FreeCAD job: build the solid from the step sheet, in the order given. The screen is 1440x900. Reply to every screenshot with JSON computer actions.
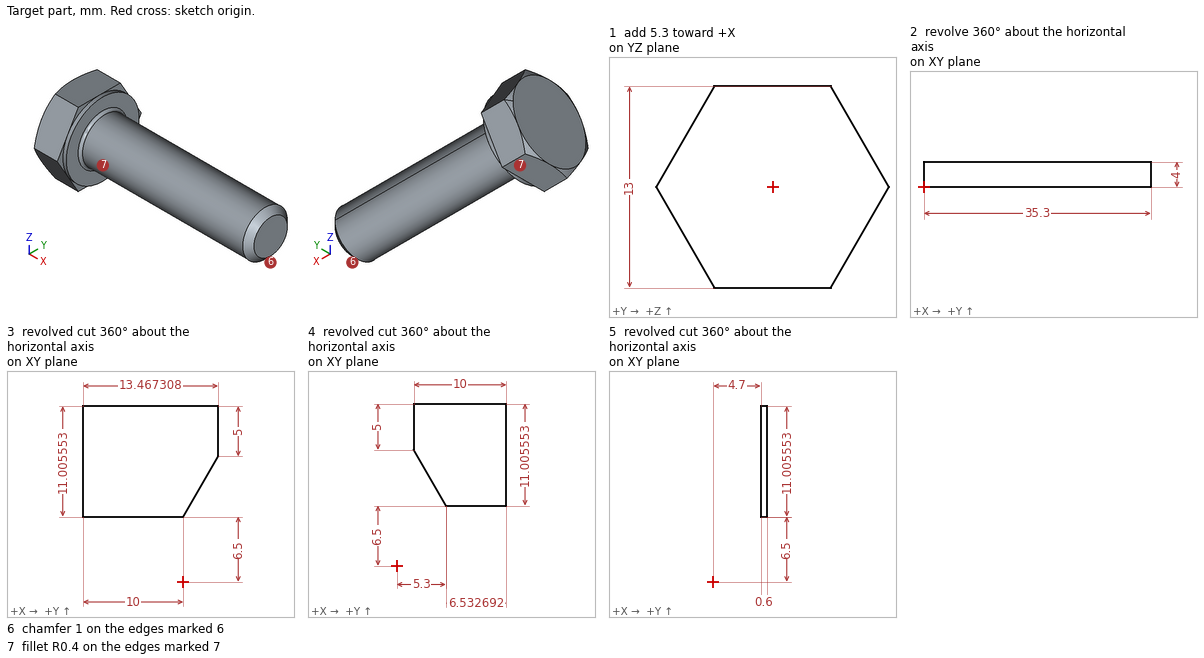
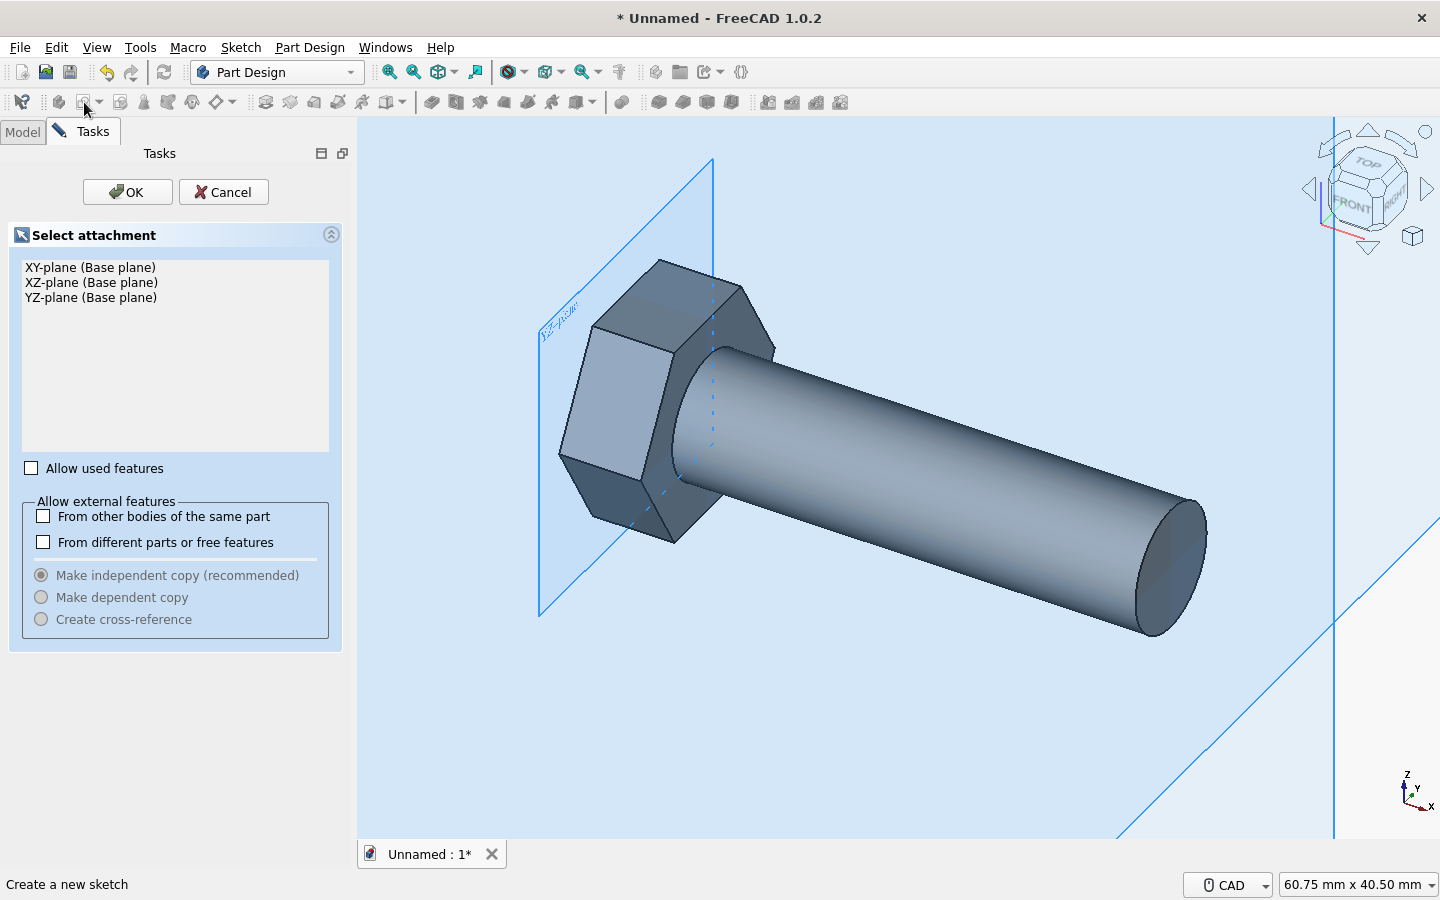
{"action": "left_click", "coordinate": [82, 268]}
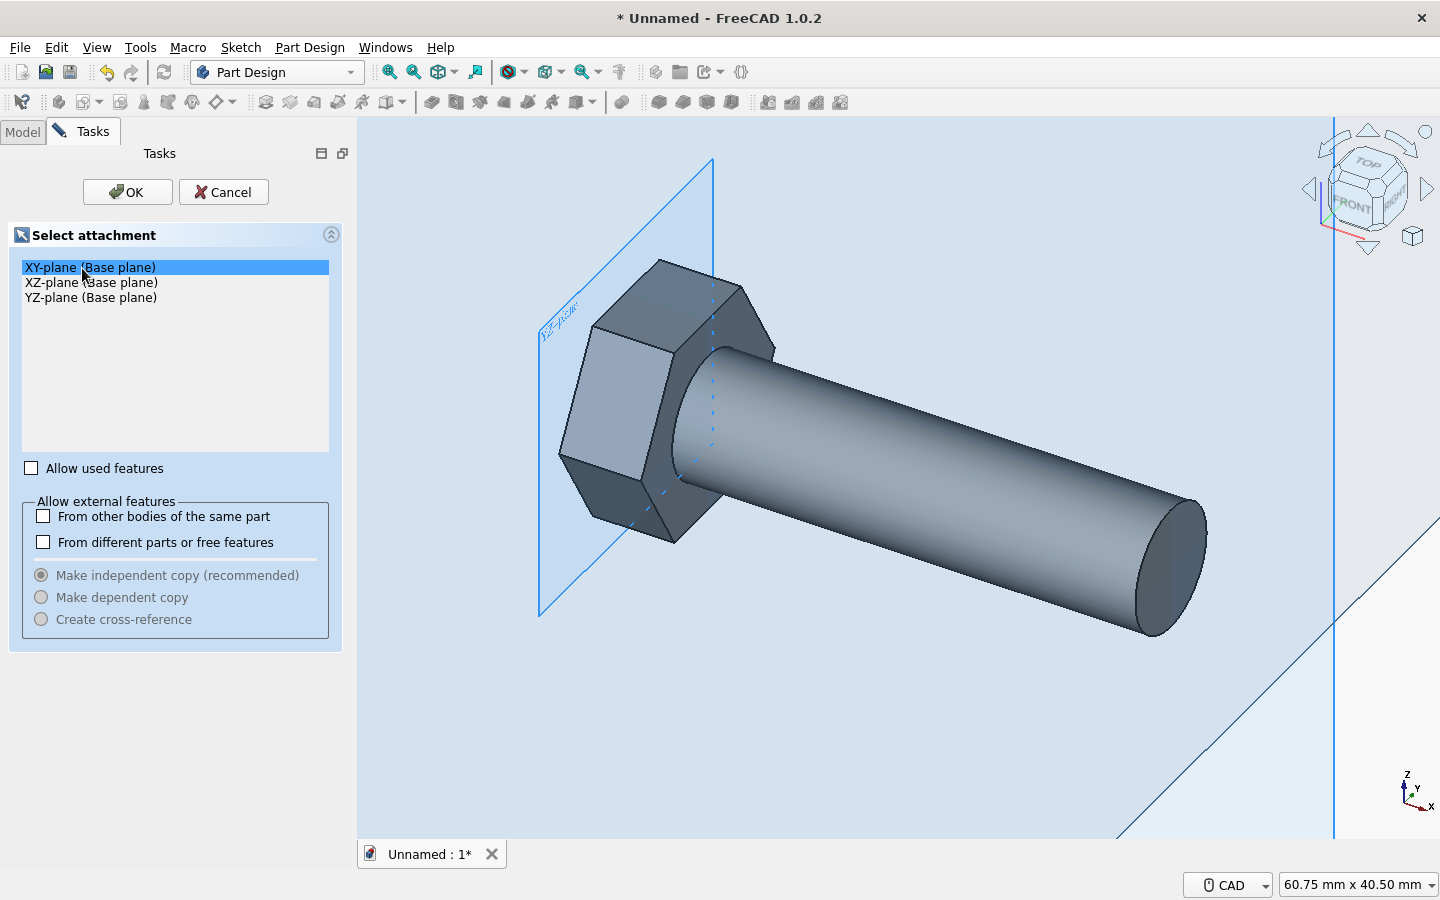
{"action": "left_click", "coordinate": [128, 192]}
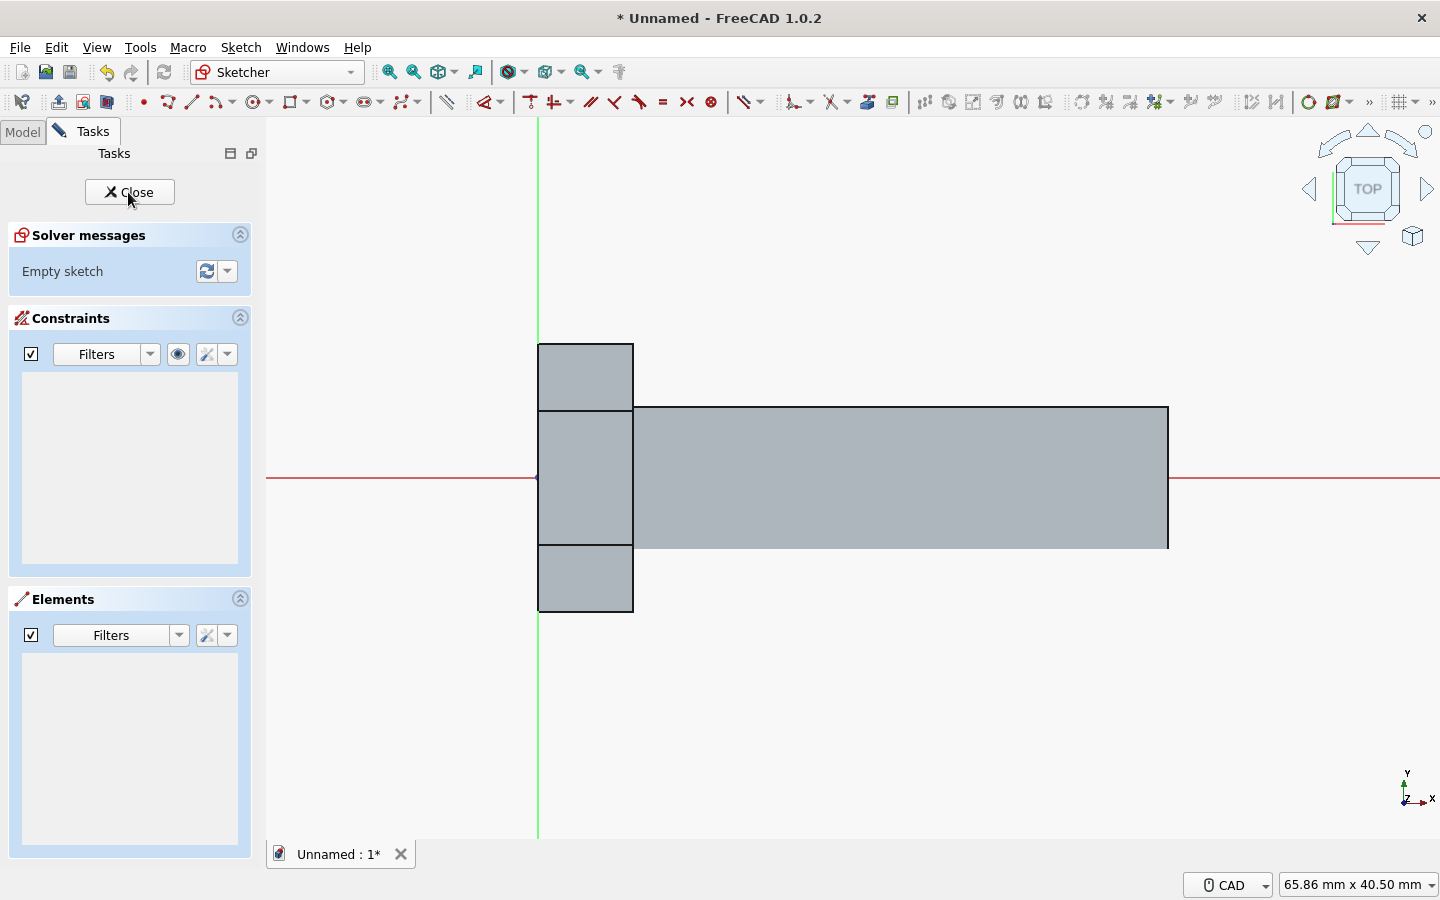
{"action": "key", "text": "q s"}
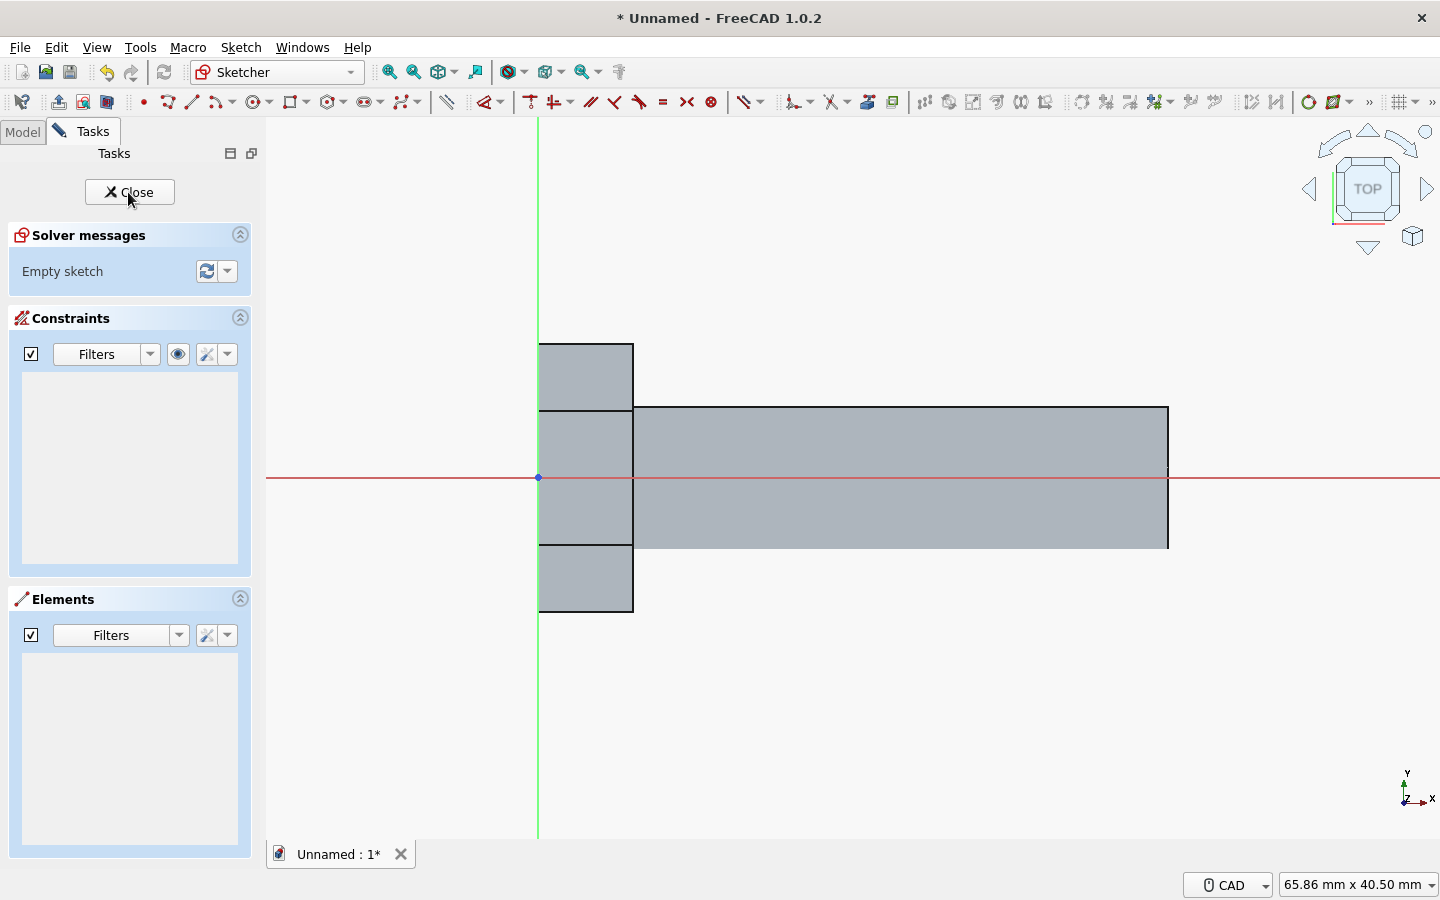
{"action": "scroll", "coordinate": [294, 145], "scroll_direction": "up", "scroll_amount": 2}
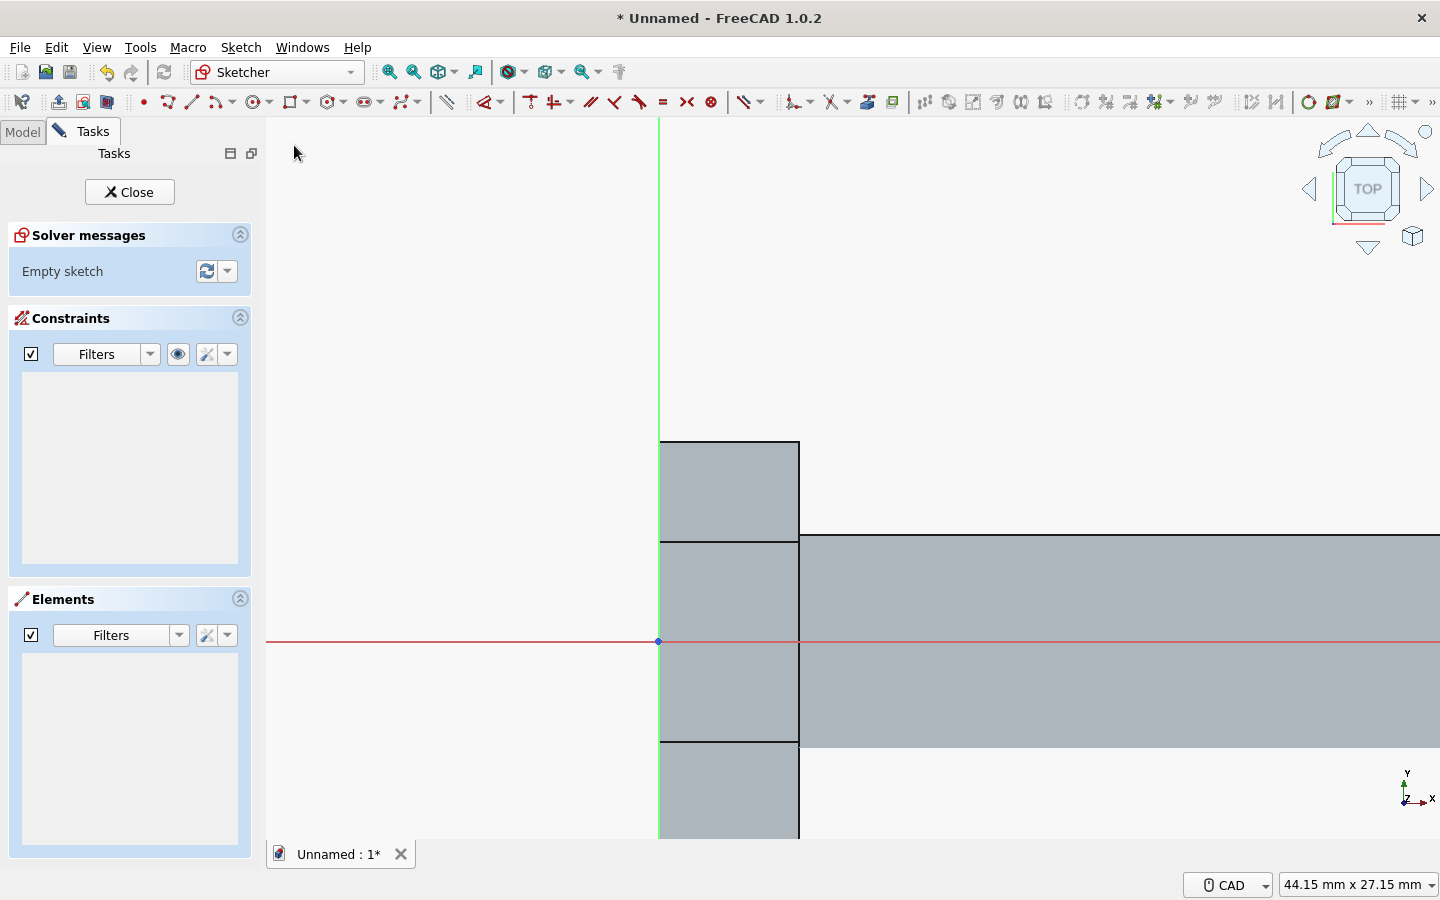
{"action": "key", "text": "g m"}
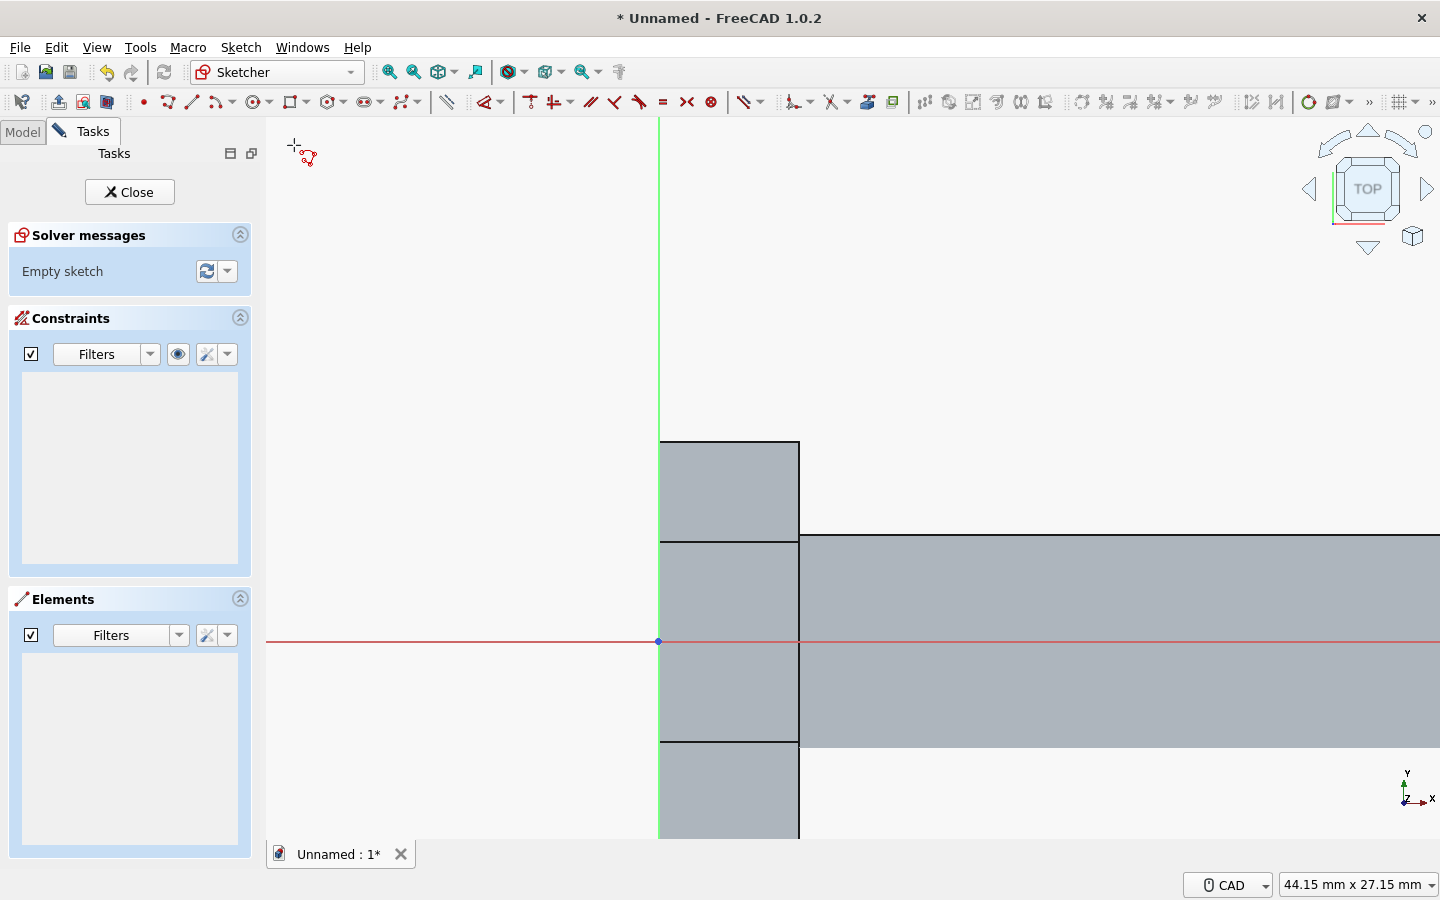
{"action": "left_click", "coordinate": [659, 469]}
{"action": "left_click", "coordinate": [751, 309]}
{"action": "left_click", "coordinate": [751, 176]}
{"action": "left_click", "coordinate": [393, 176]}
{"action": "left_click", "coordinate": [393, 469]}
{"action": "left_click", "coordinate": [659, 470]}
{"action": "key", "text": "Escape"}
{"action": "key", "text": "Escape"}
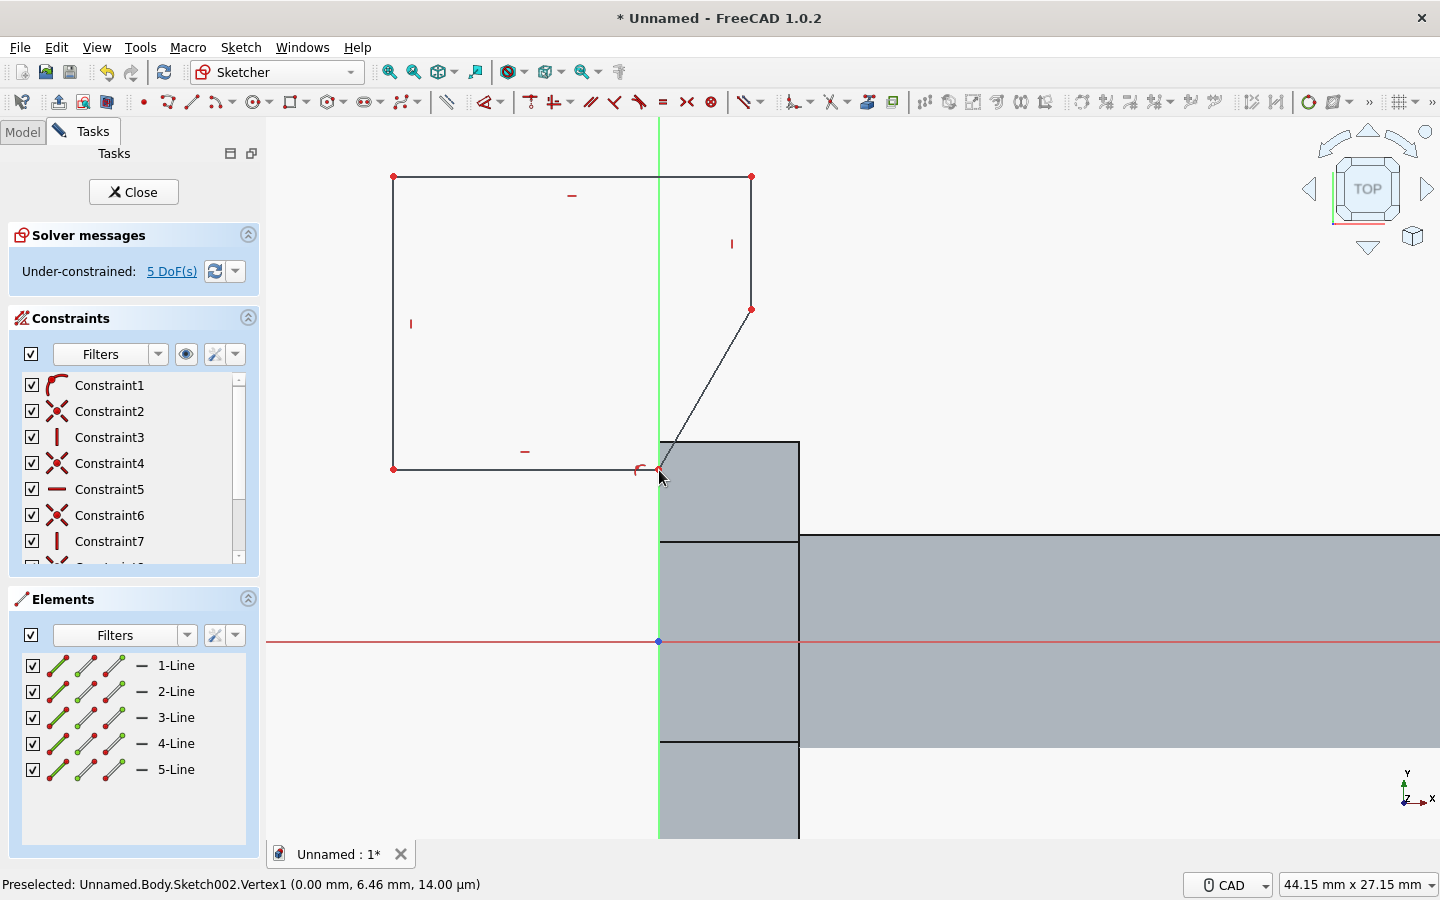
{"action": "left_click", "coordinate": [484, 102]}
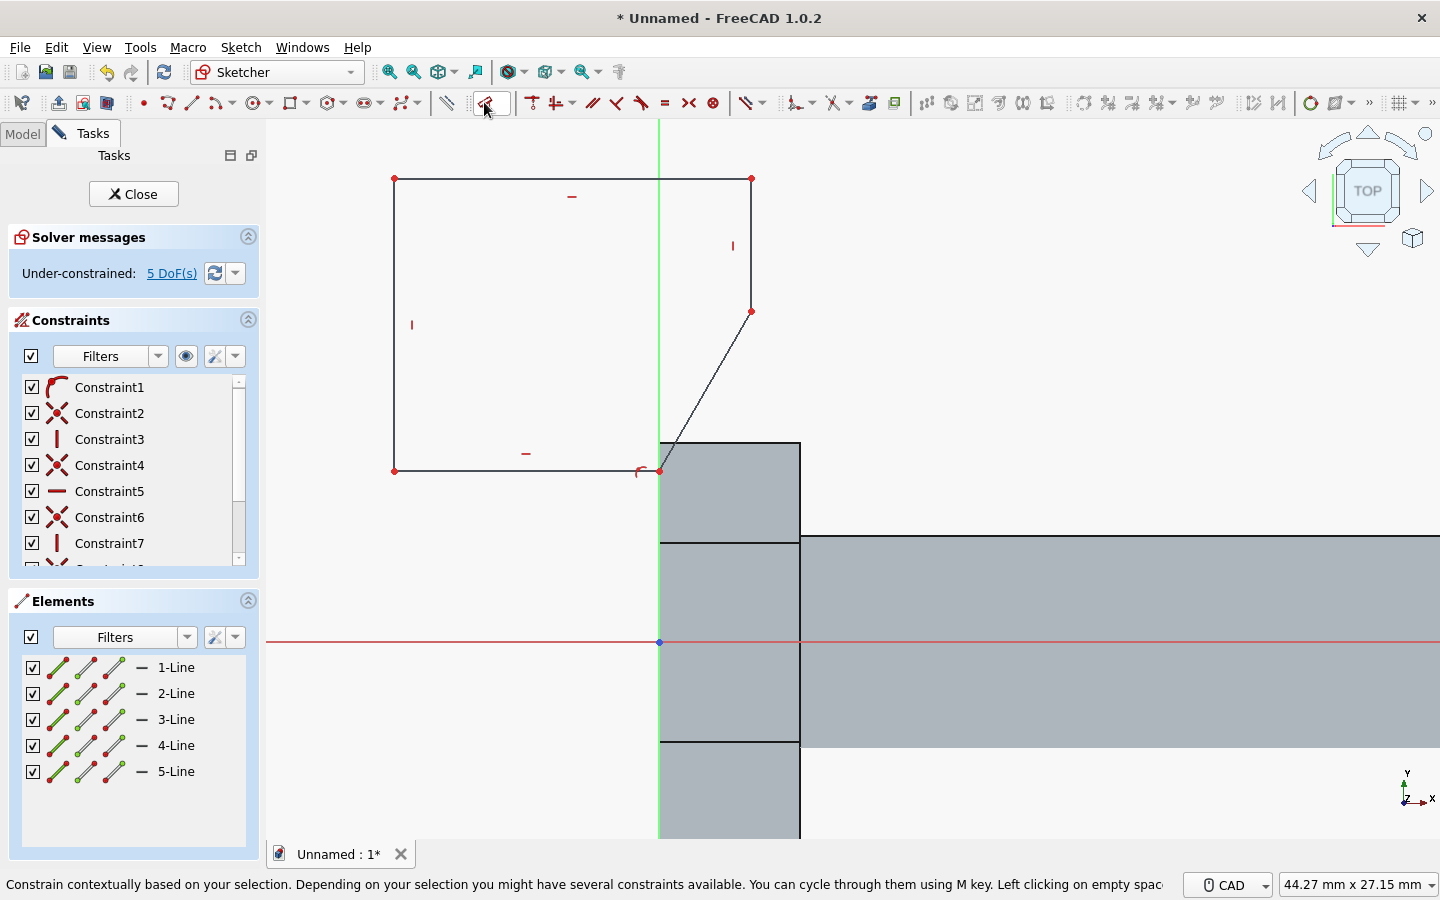
{"action": "left_click", "coordinate": [751, 272]}
{"action": "left_click", "coordinate": [785, 245]}